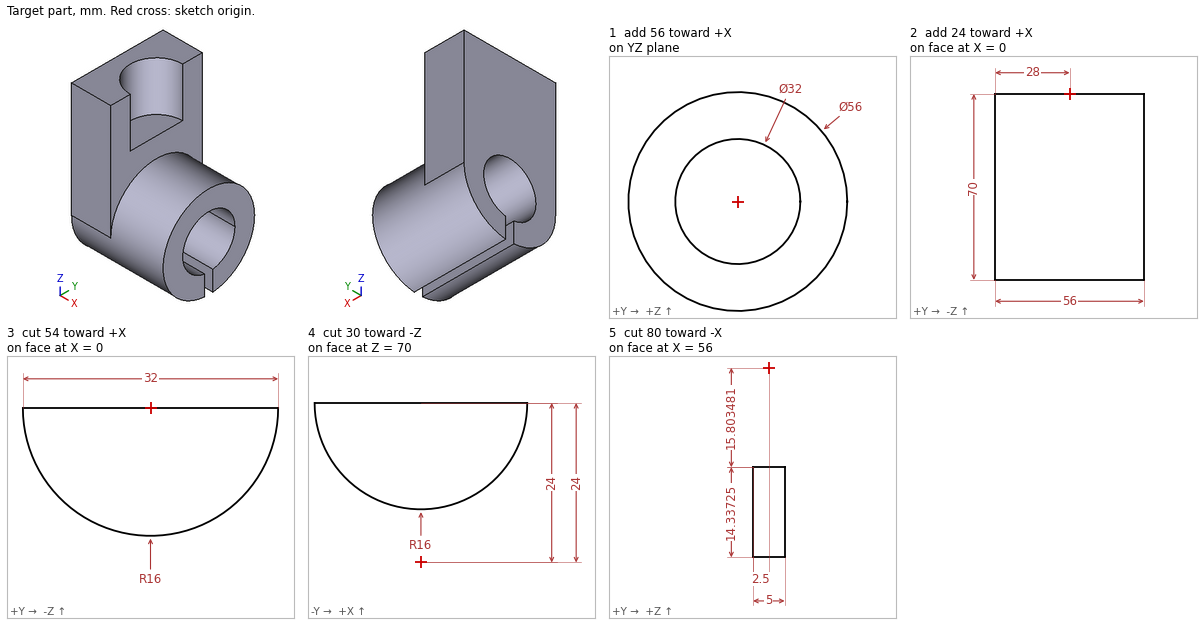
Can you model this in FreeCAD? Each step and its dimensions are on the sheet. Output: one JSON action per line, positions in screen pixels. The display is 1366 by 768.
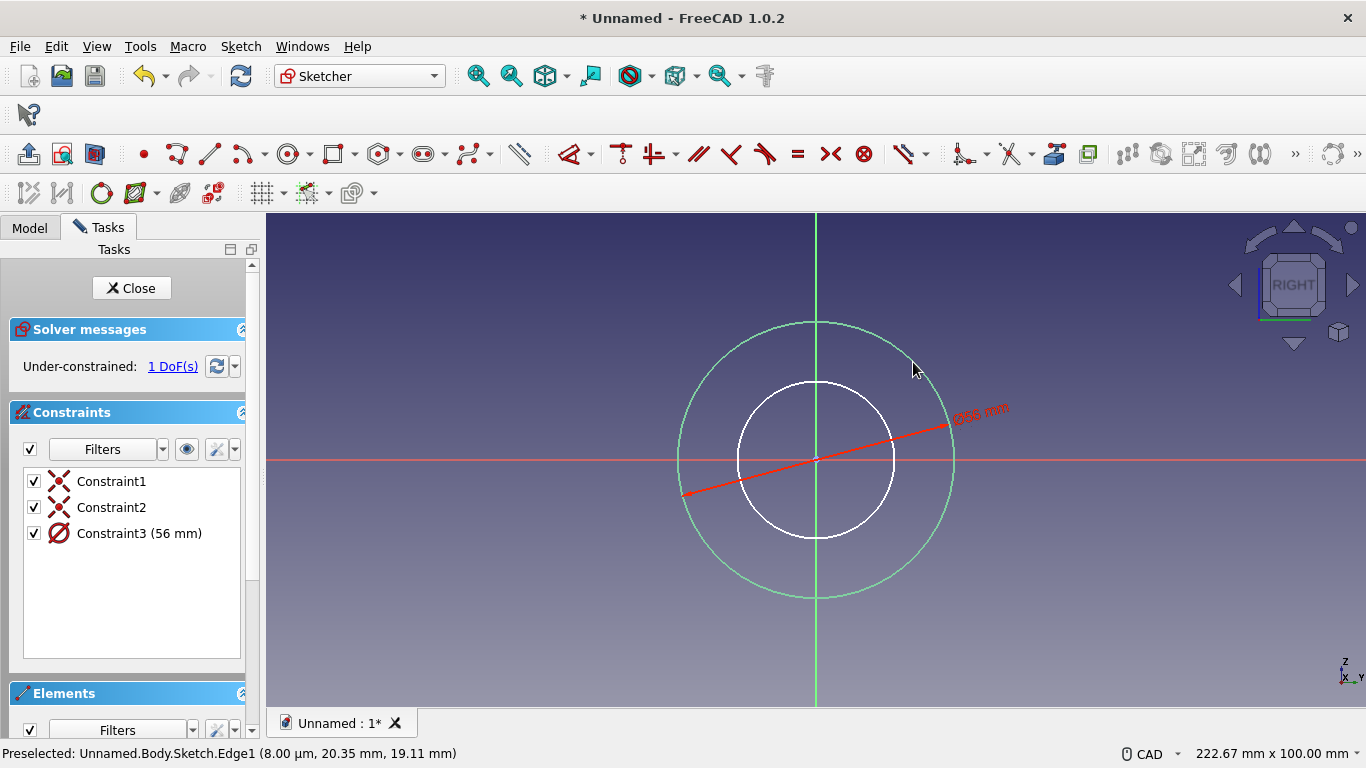
{"action": "left_click", "coordinate": [871, 404]}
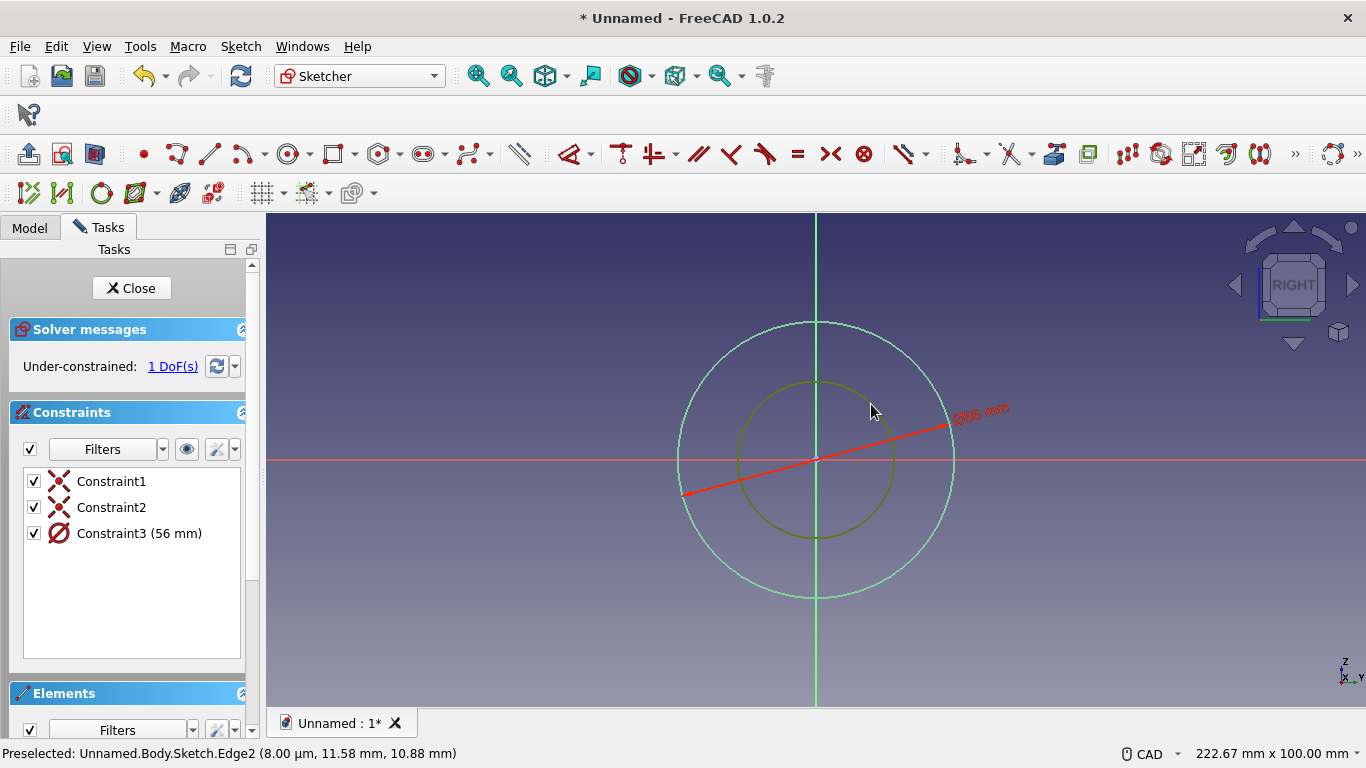
{"action": "left_click", "coordinate": [590, 154]}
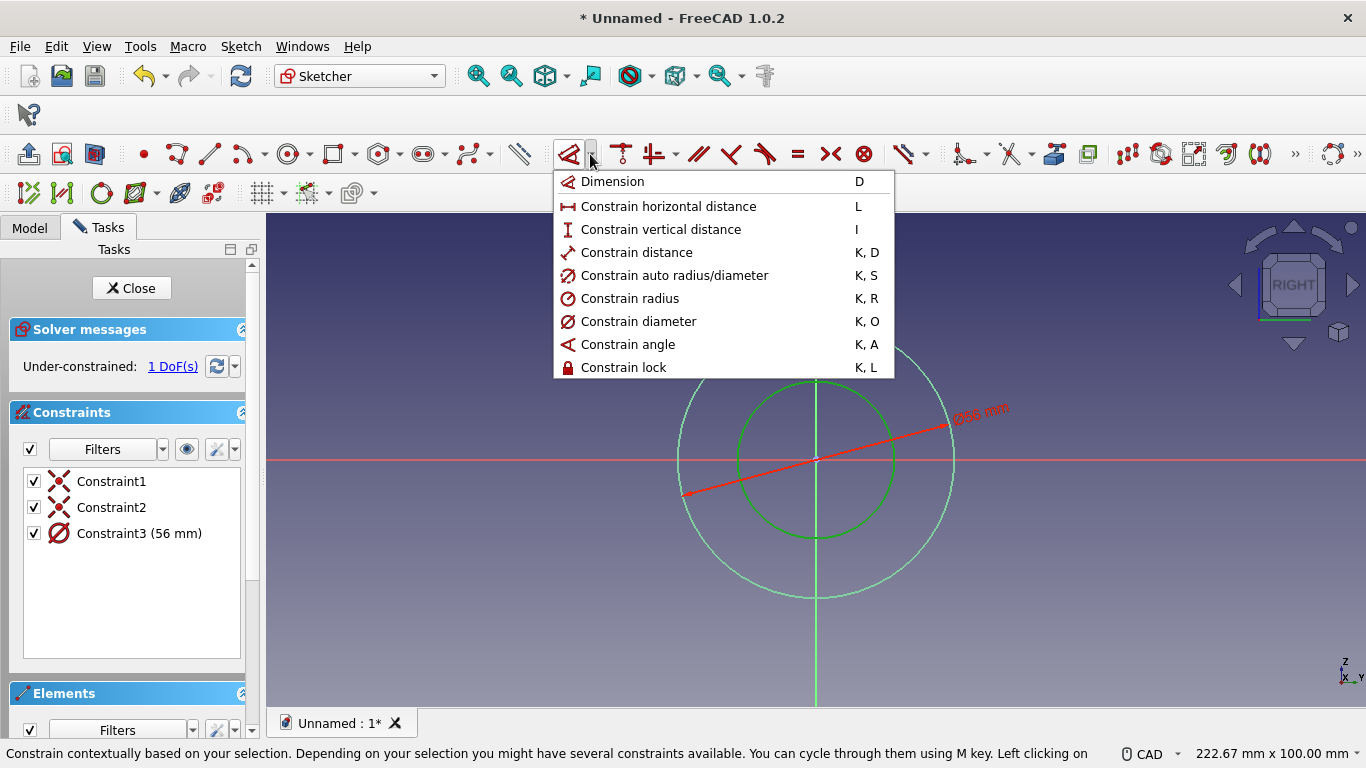
{"action": "left_click", "coordinate": [724, 322]}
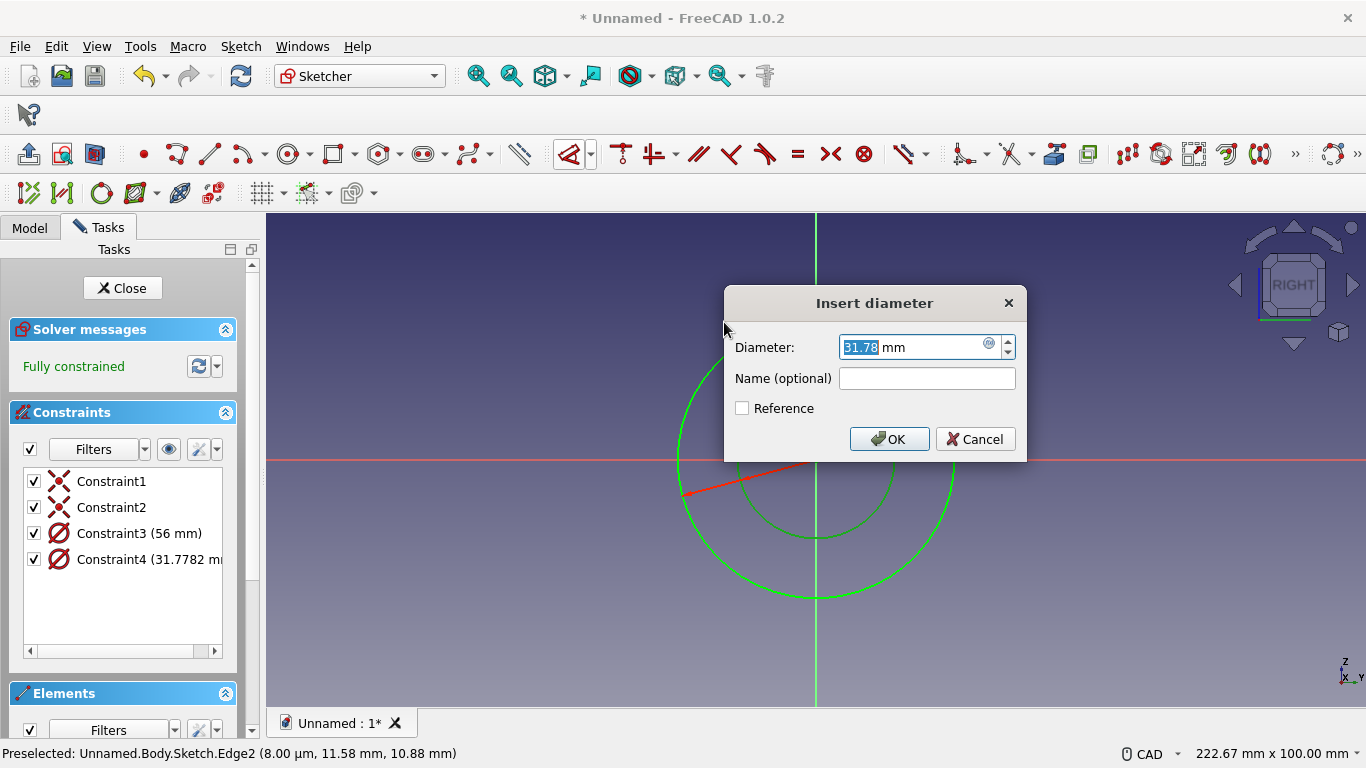
{"action": "type", "text": "32"}
{"action": "key", "text": "Return"}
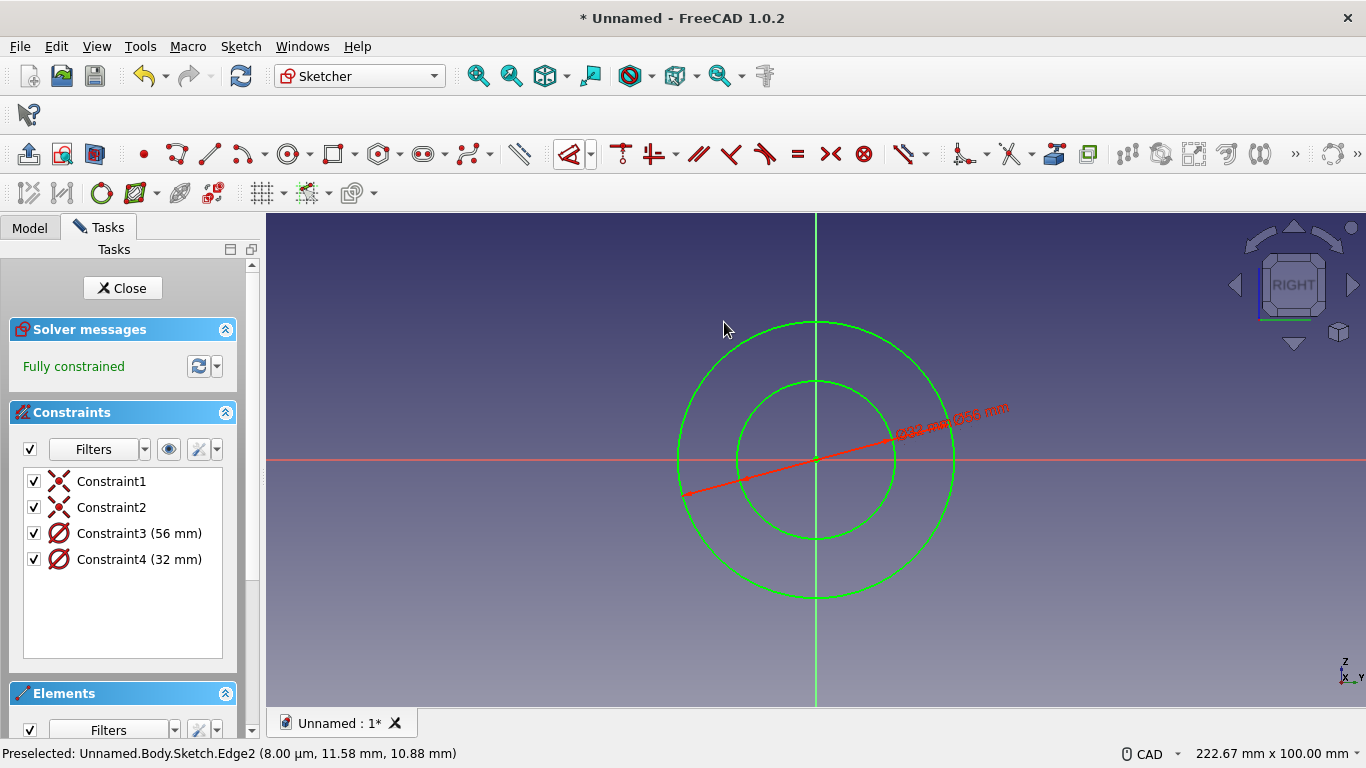
{"action": "left_click", "coordinate": [123, 288]}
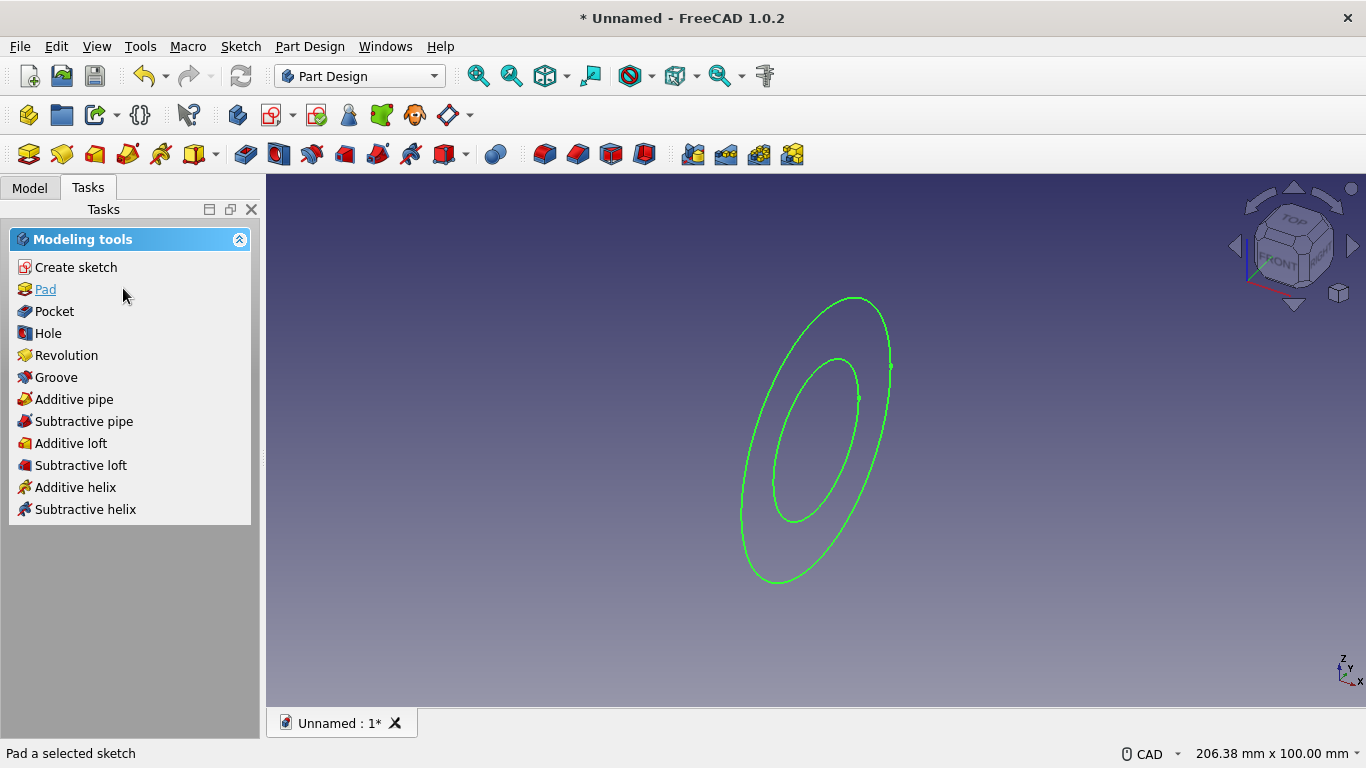
{"action": "left_click", "coordinate": [29, 154]}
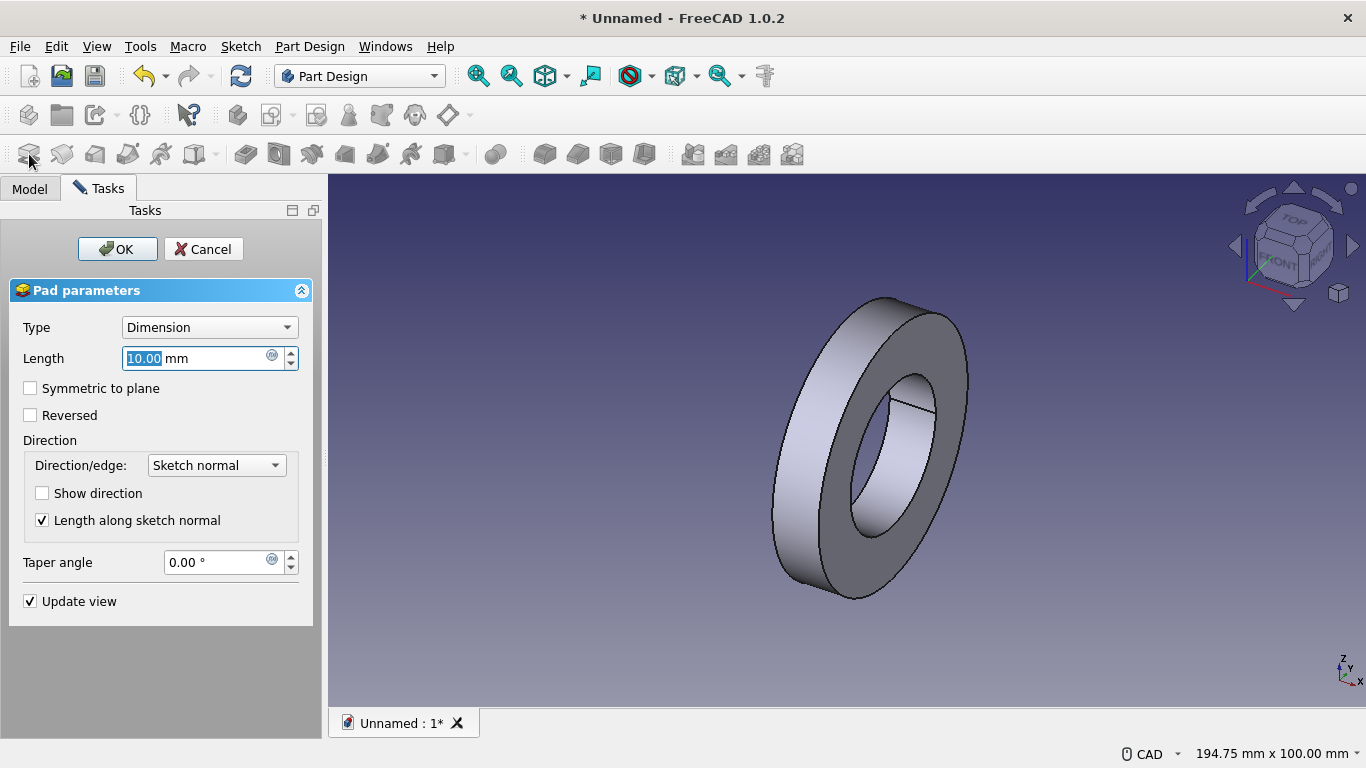
{"action": "type", "text": "56"}
{"action": "key", "text": "Tab"}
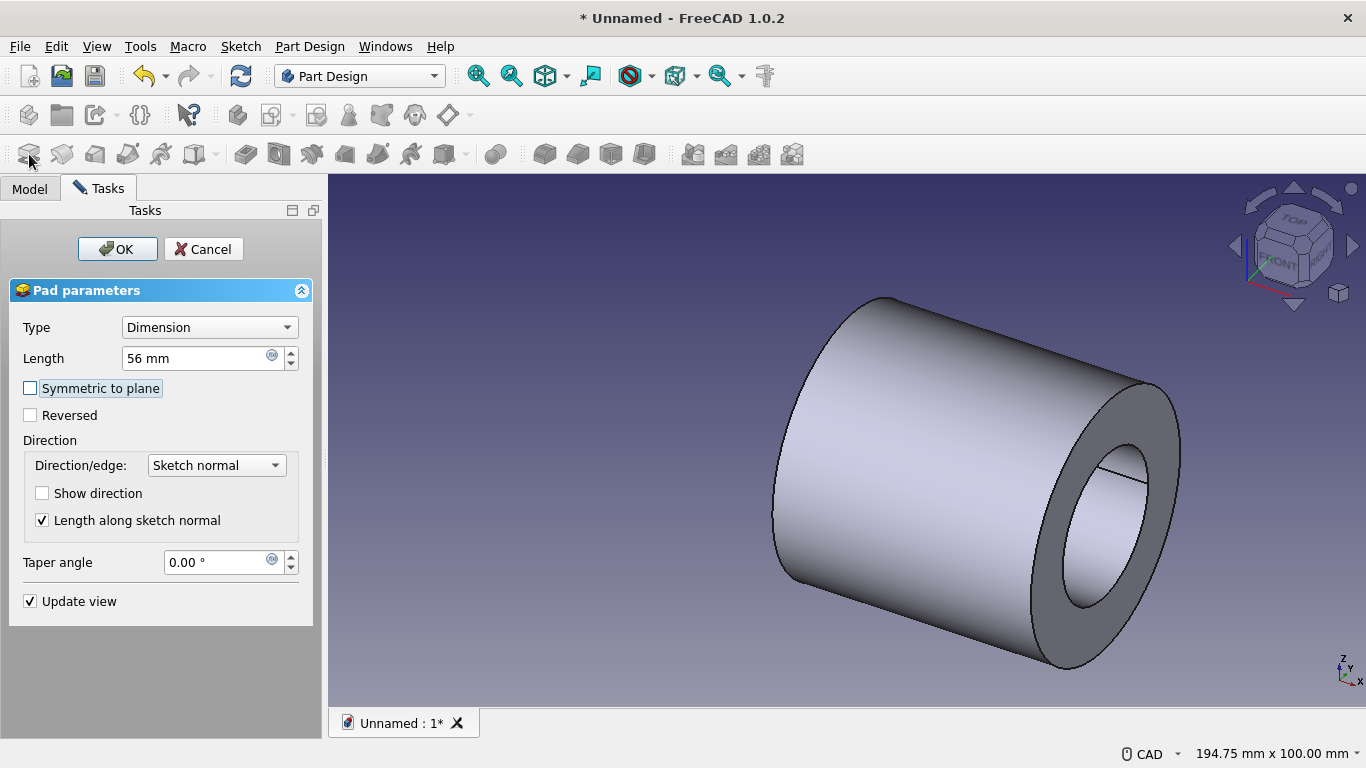
{"action": "left_click", "coordinate": [118, 249]}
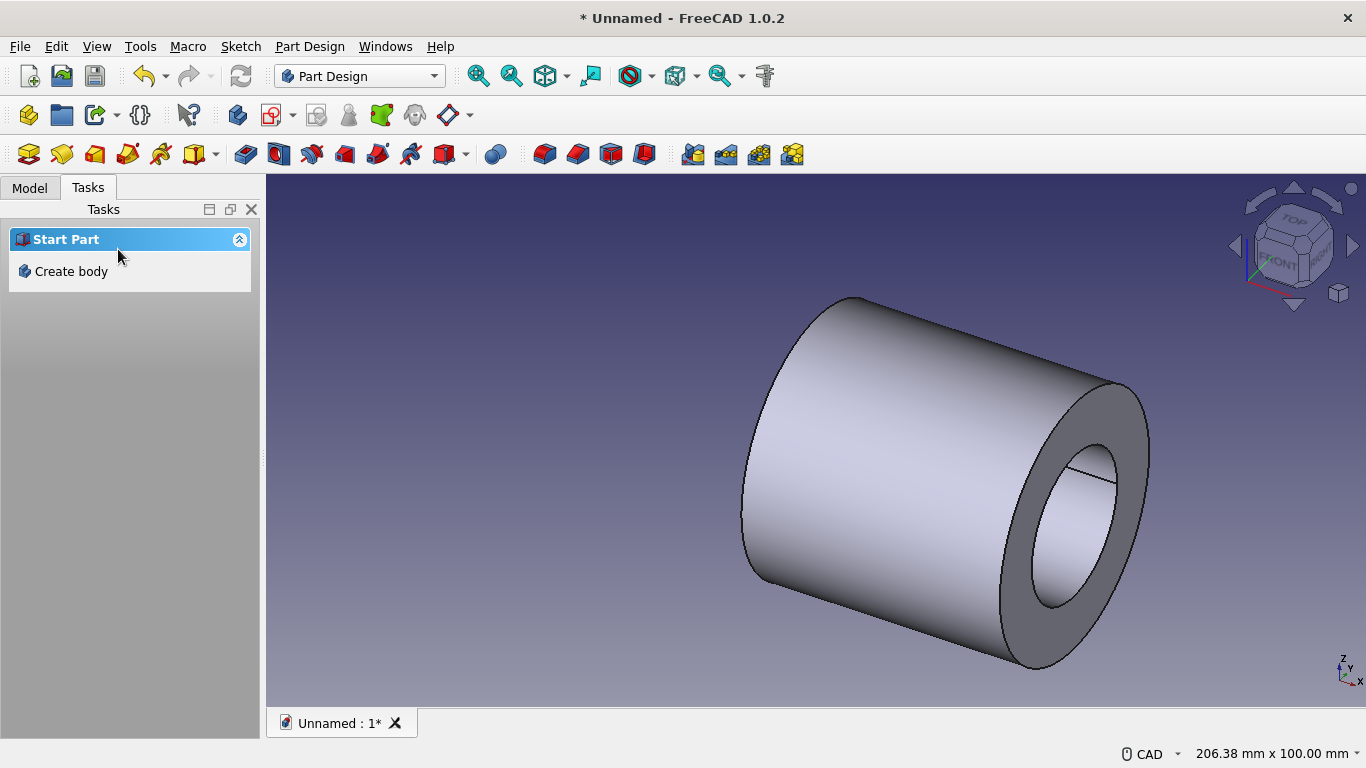
{"action": "left_click", "coordinate": [479, 76]}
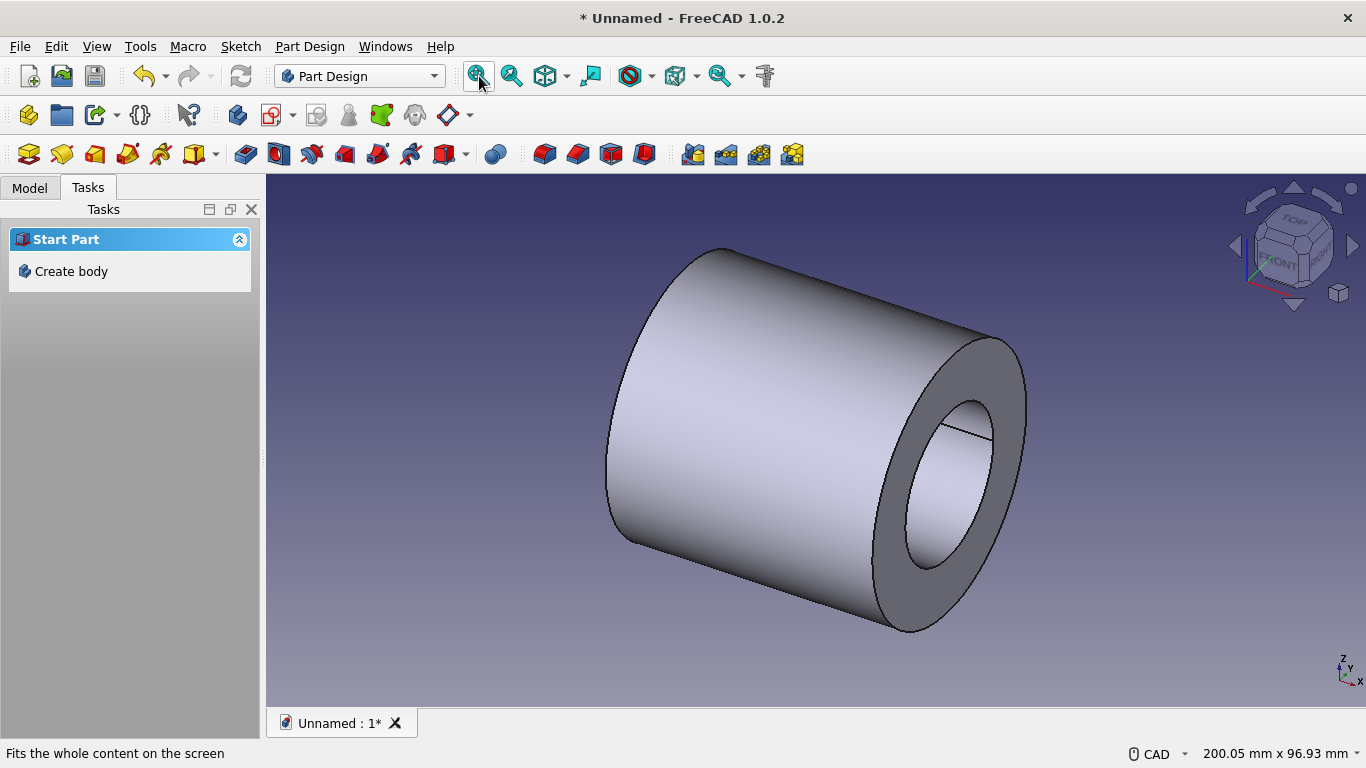
{"action": "key", "text": "6"}